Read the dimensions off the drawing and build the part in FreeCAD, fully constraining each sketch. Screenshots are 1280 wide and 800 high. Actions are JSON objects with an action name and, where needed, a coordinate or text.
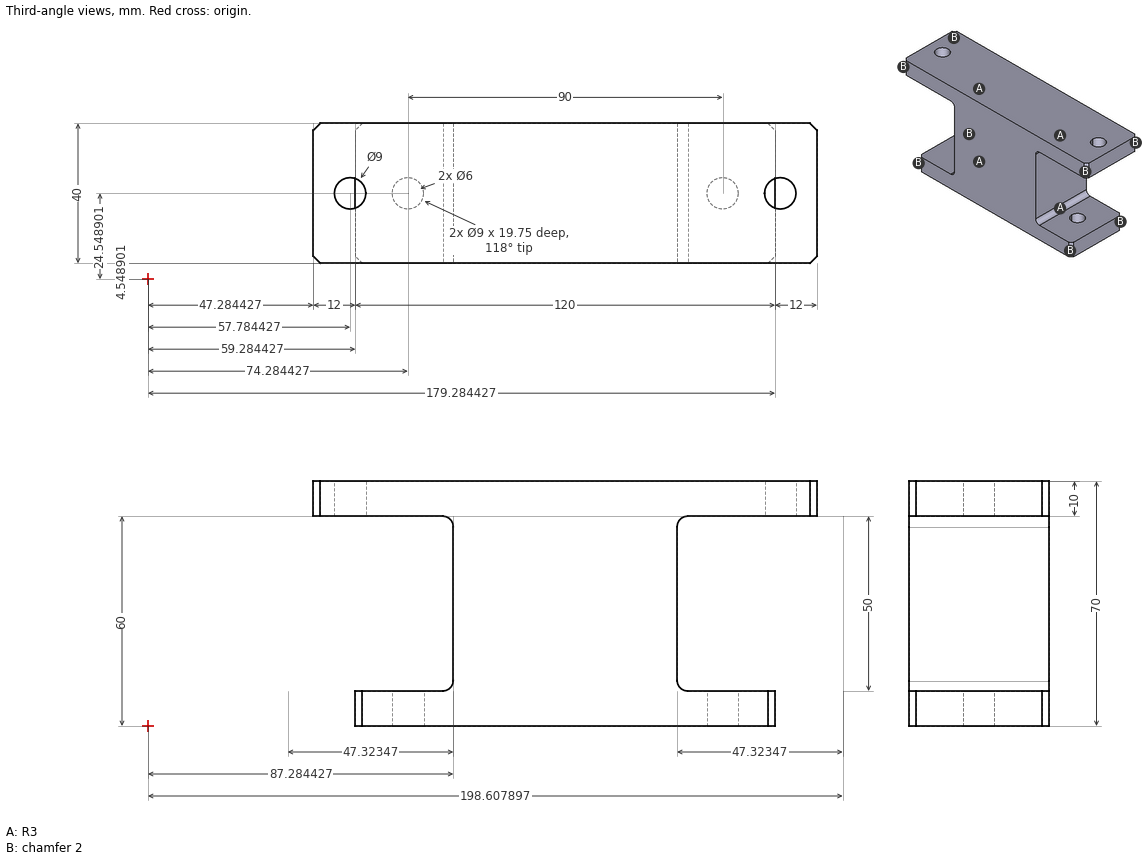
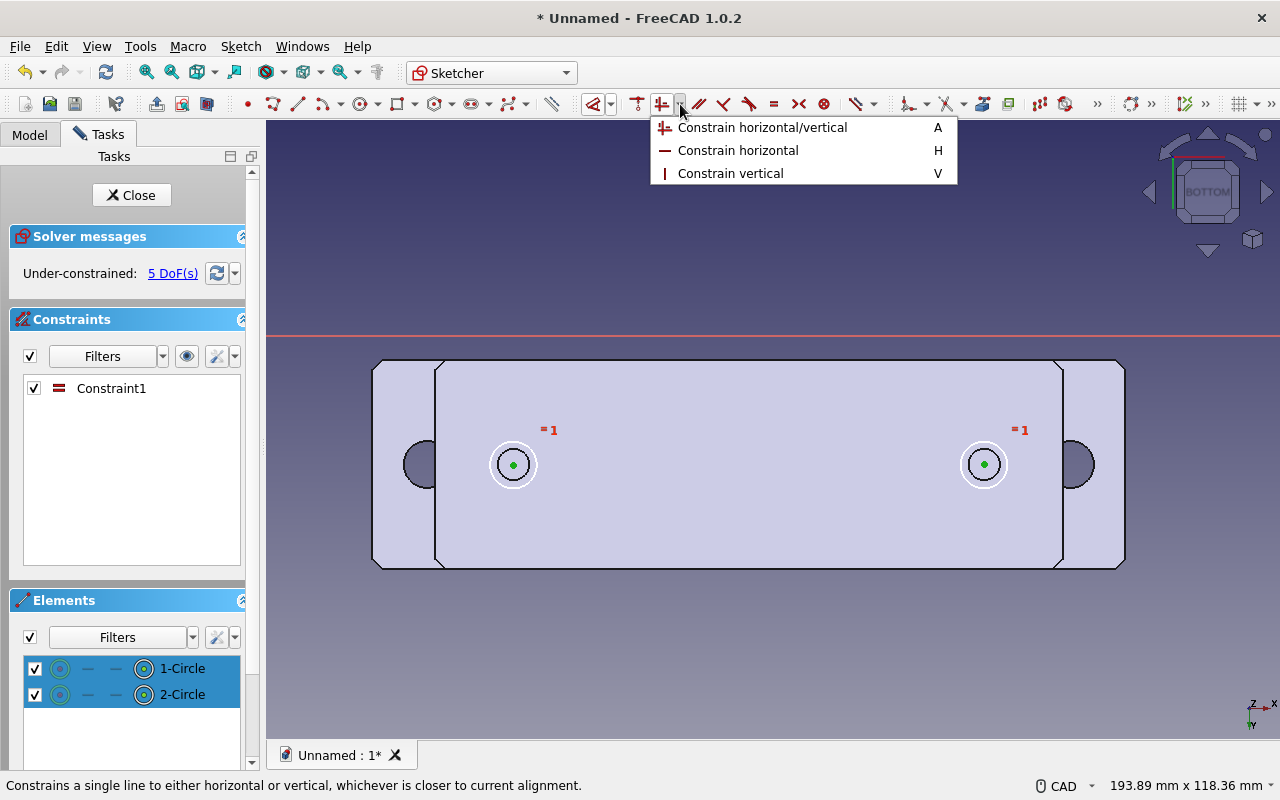
{"action": "left_click", "coordinate": [804, 150]}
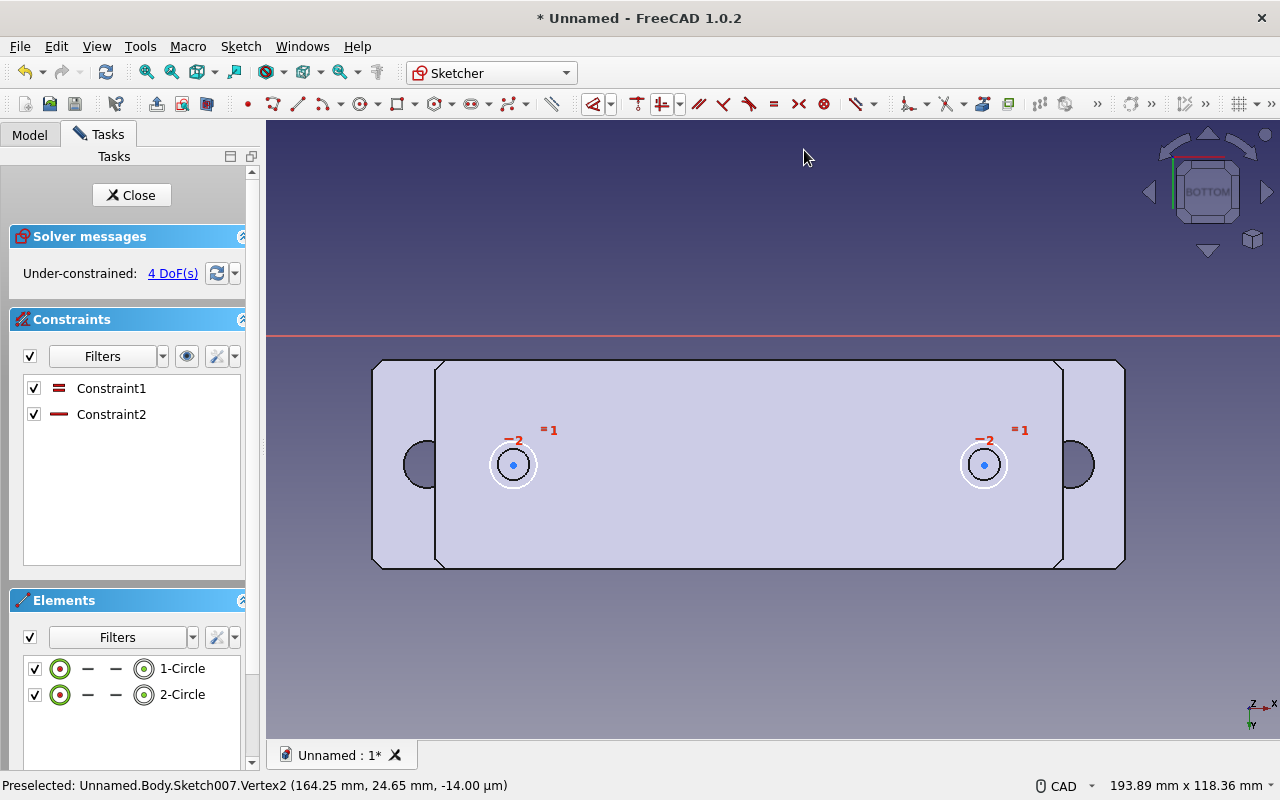
{"action": "left_click", "coordinate": [530, 448]}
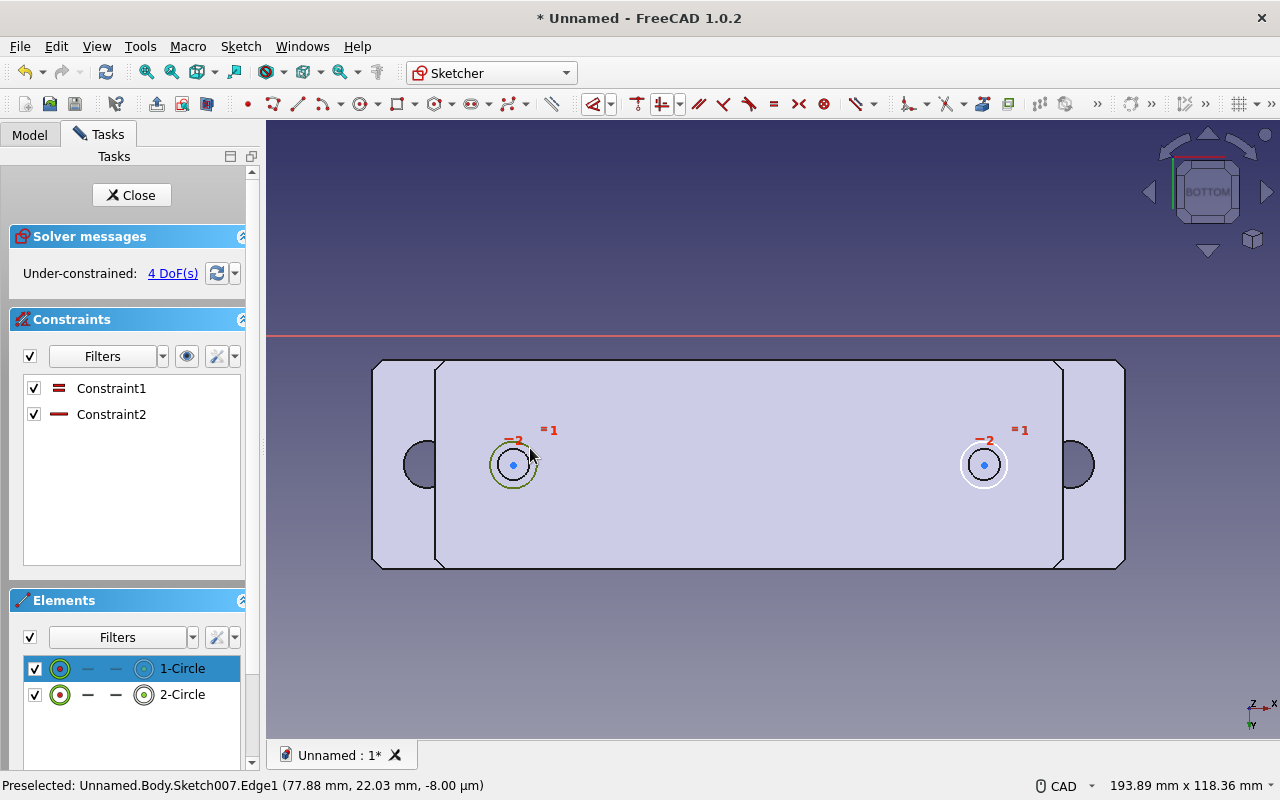
{"action": "key", "text": "k o"}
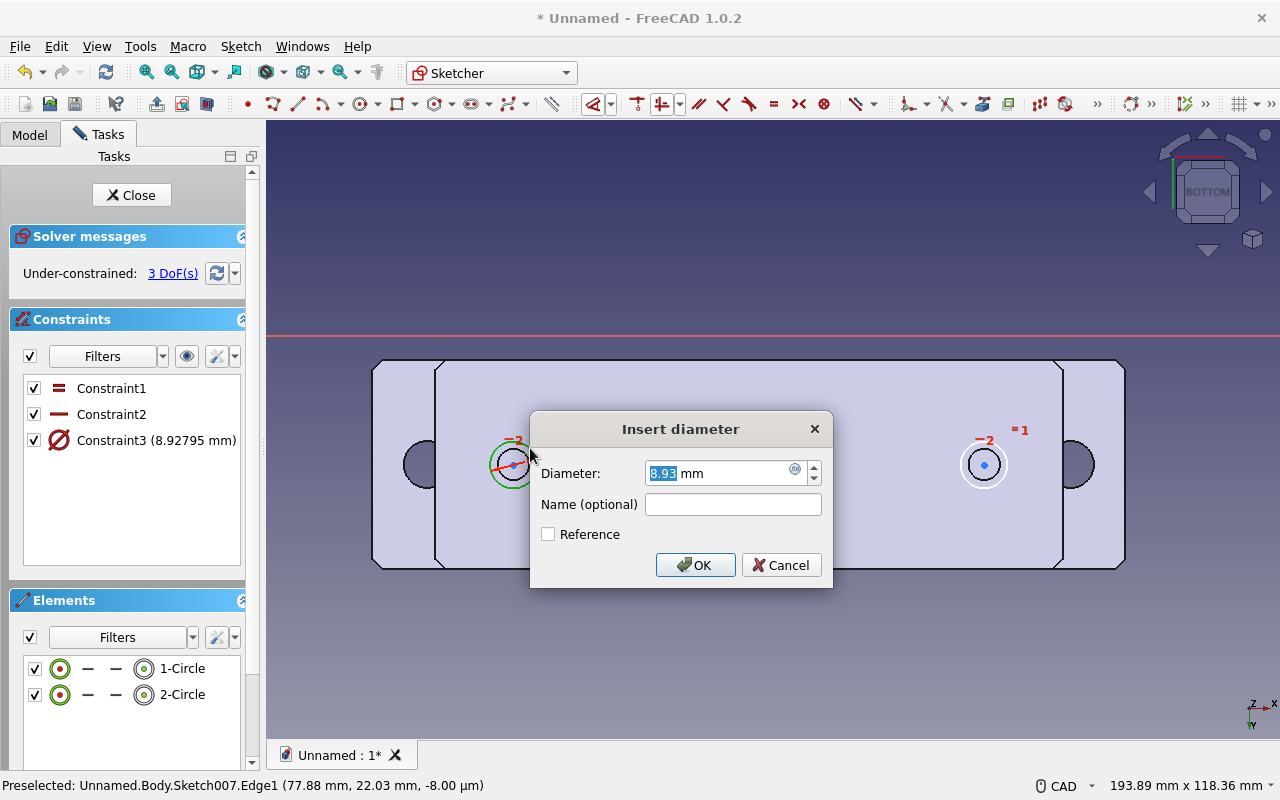
{"action": "type", "text": "9"}
{"action": "key", "text": "Return"}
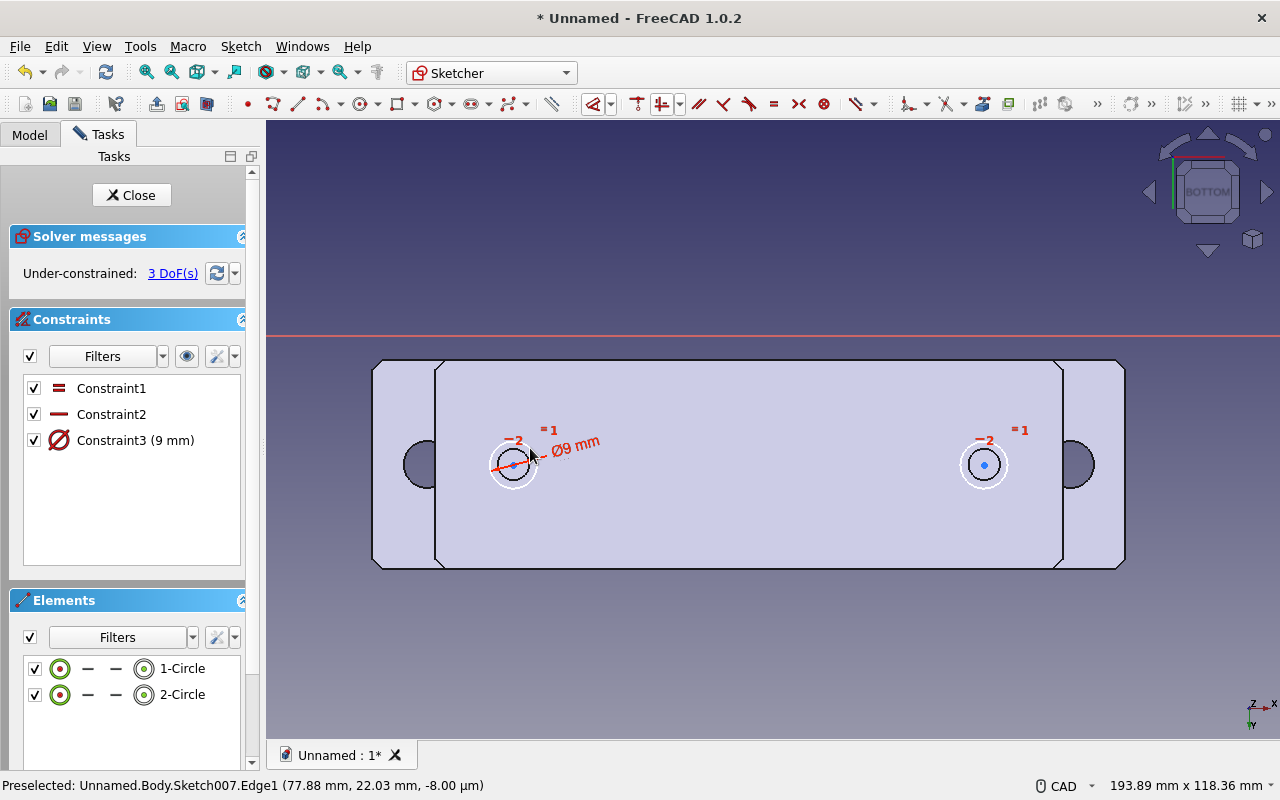
{"action": "left_click", "coordinate": [513, 465]}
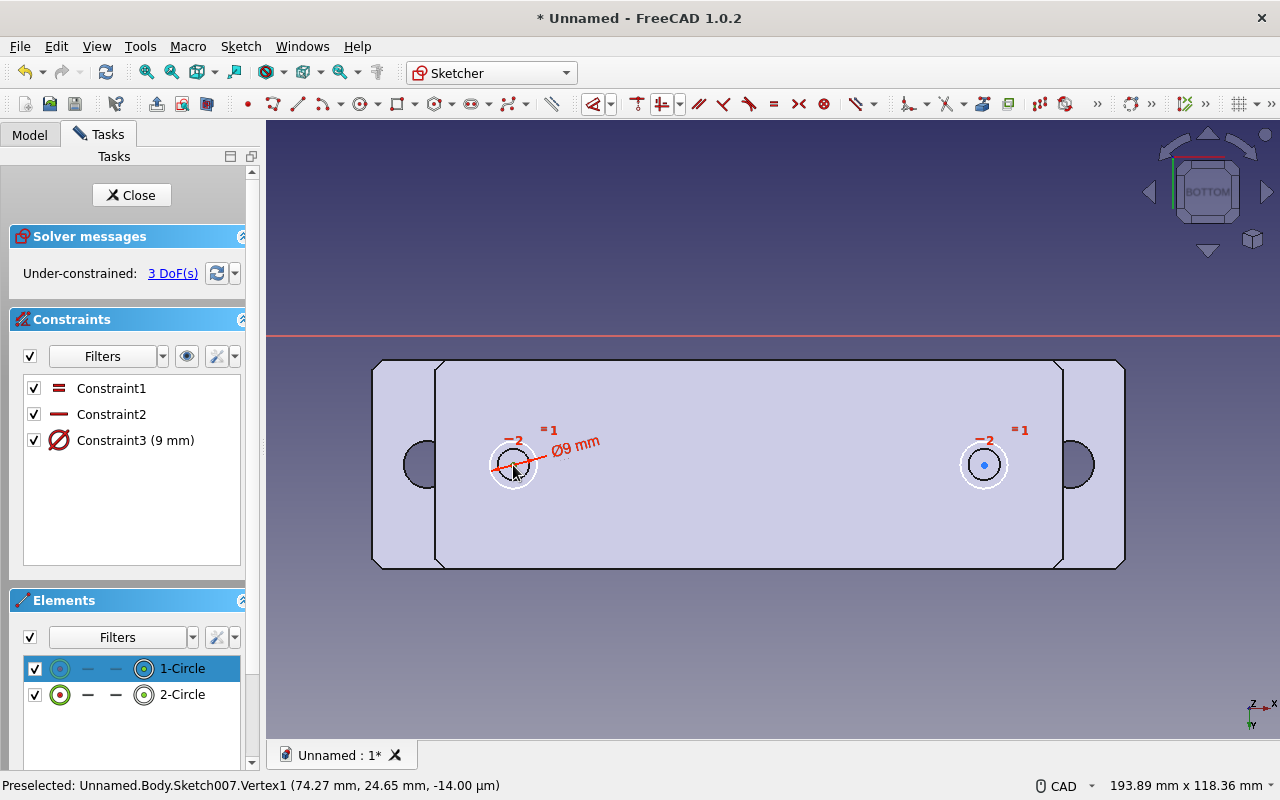
{"action": "left_click", "coordinate": [984, 465]}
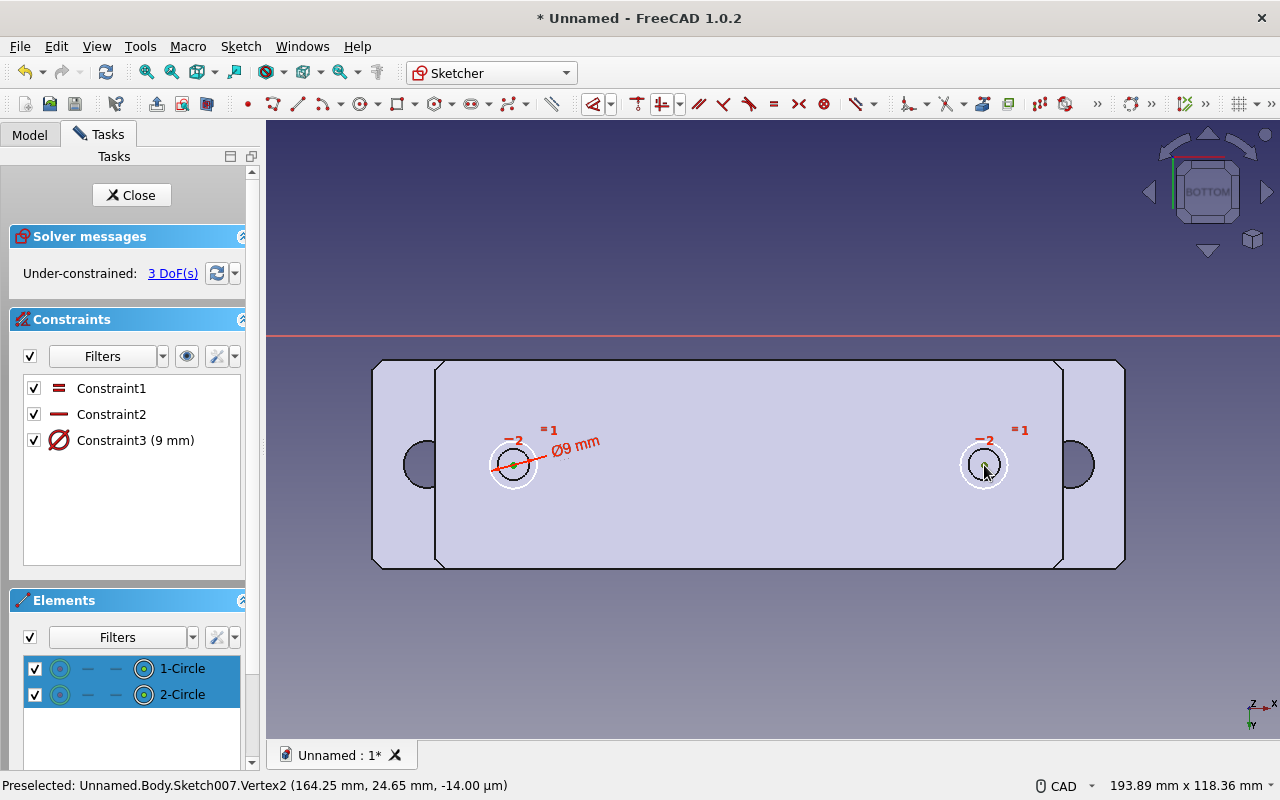
{"action": "key", "text": "l"}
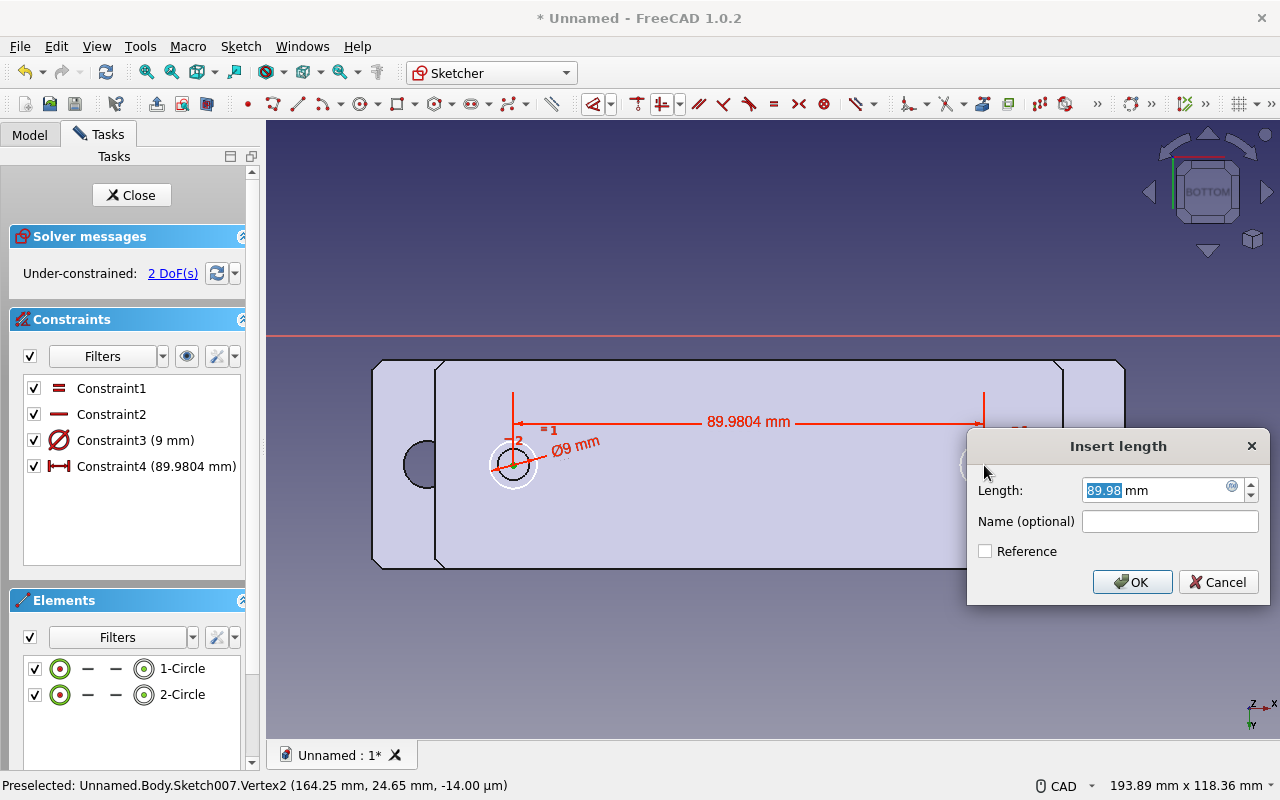
{"action": "type", "text": "90"}
{"action": "key", "text": "Return"}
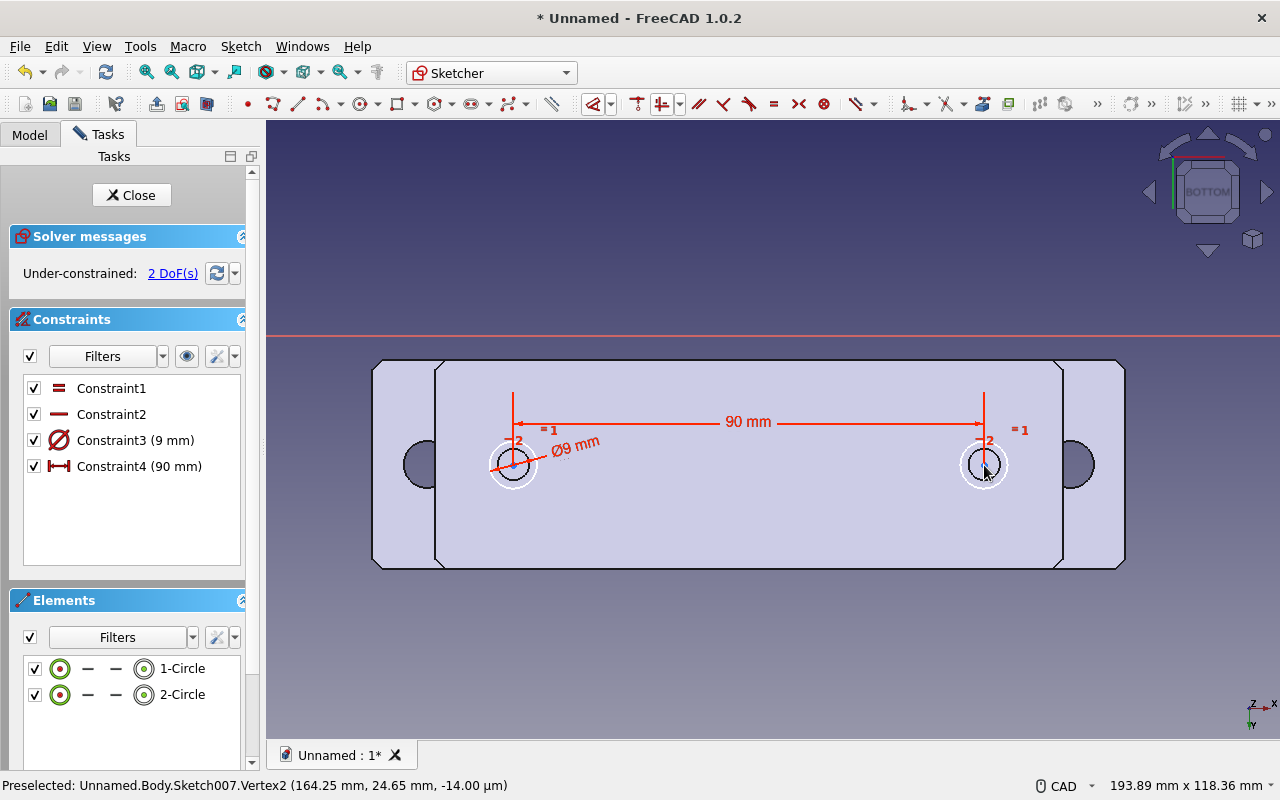
{"action": "left_click", "coordinate": [513, 465]}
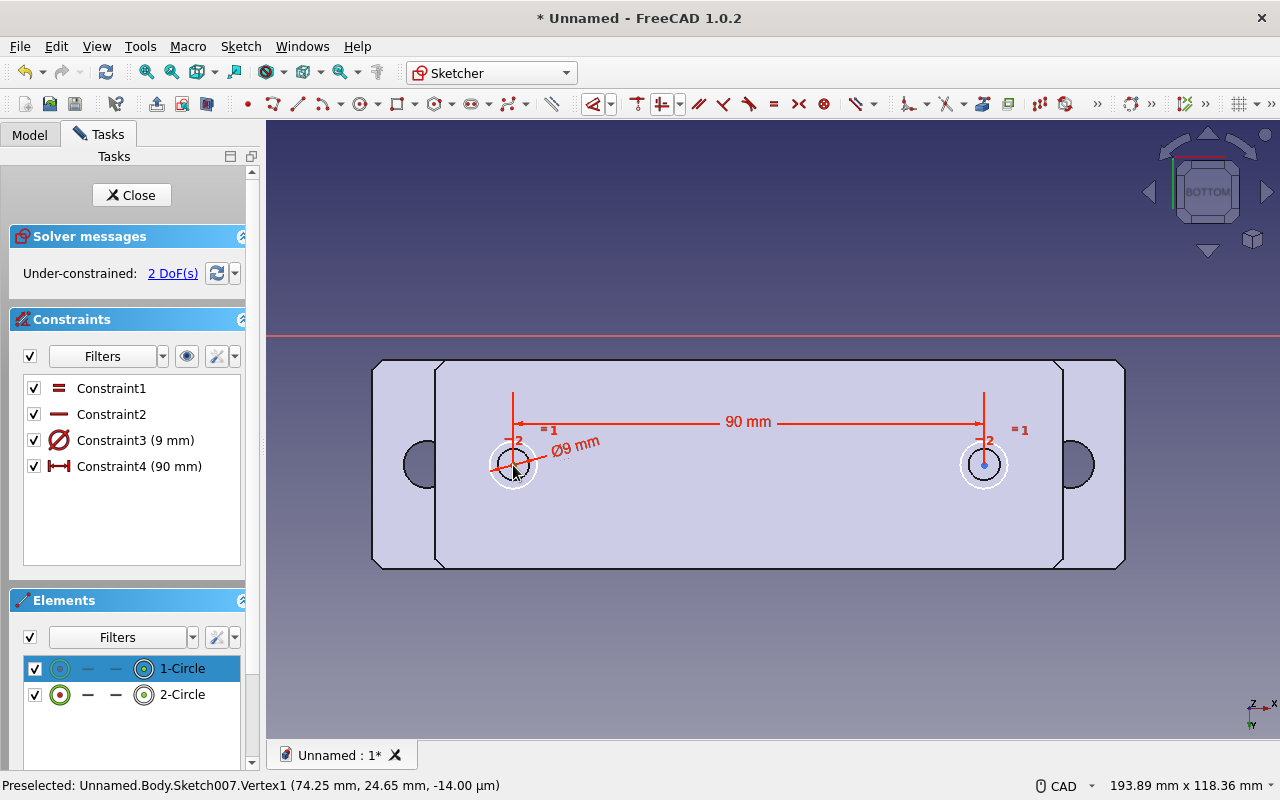
{"action": "key", "text": "l"}